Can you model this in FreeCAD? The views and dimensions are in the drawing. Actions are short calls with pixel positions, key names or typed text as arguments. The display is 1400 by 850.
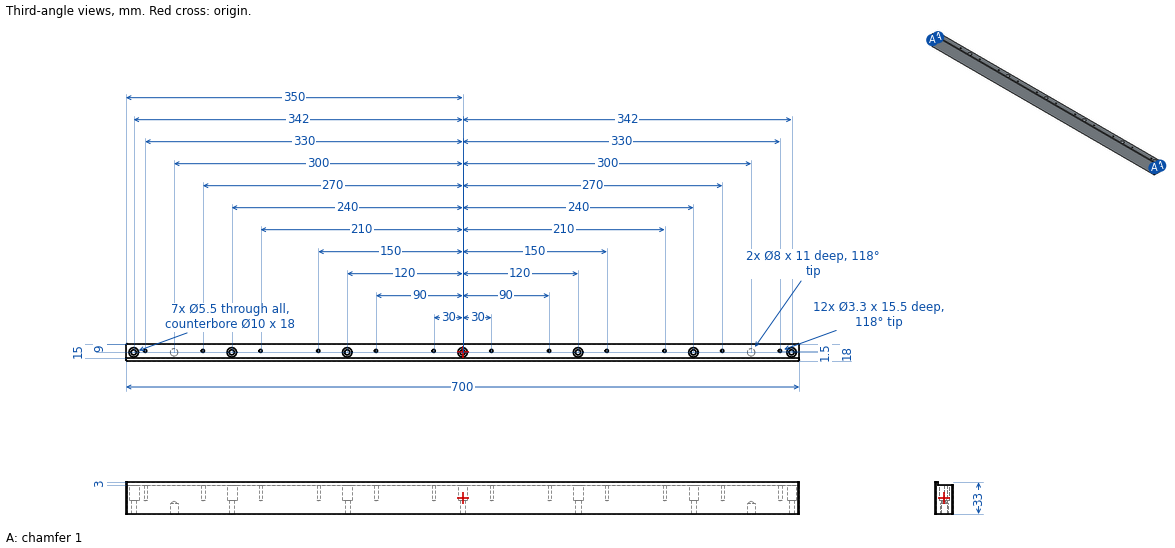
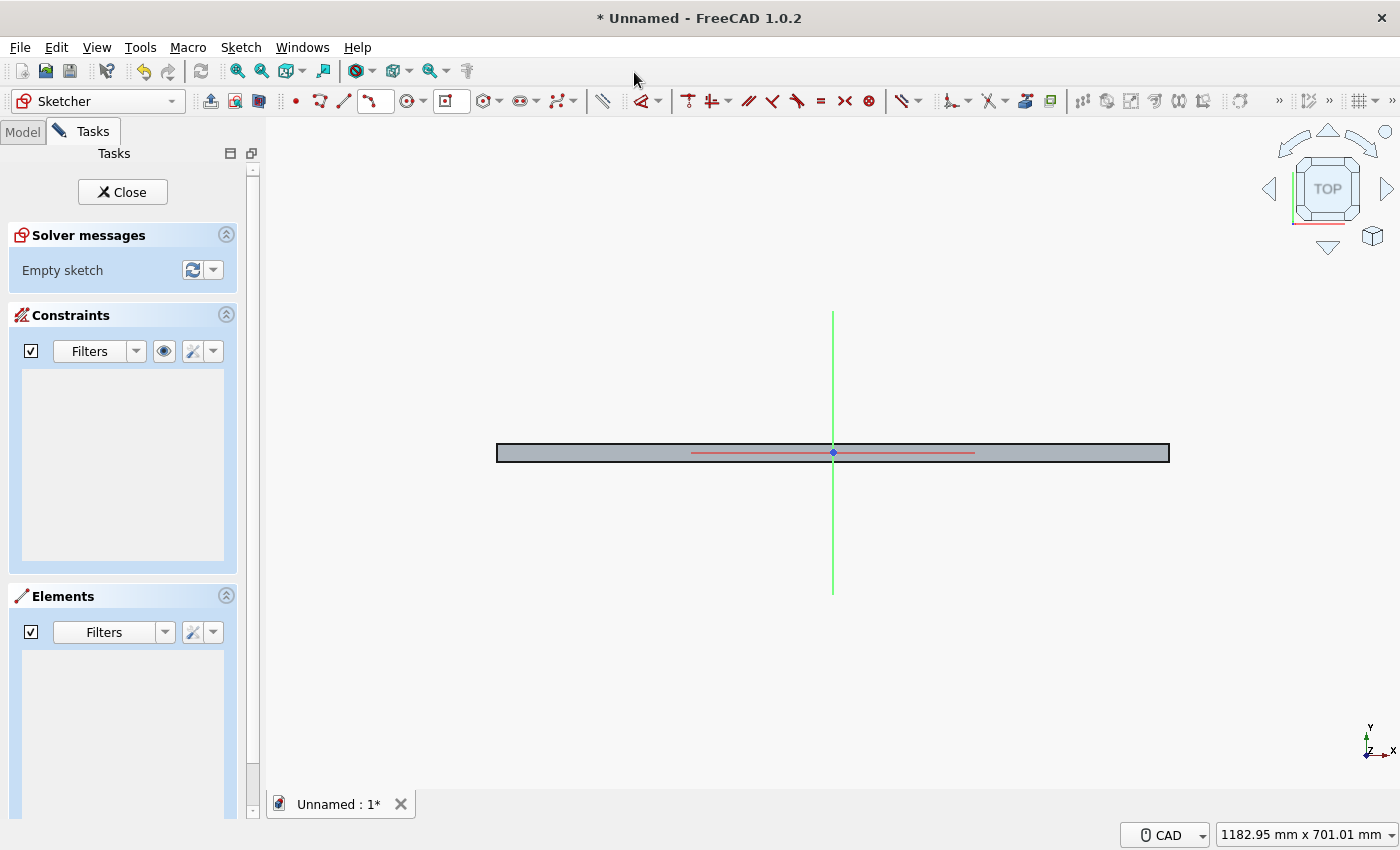
key(g)
key(r)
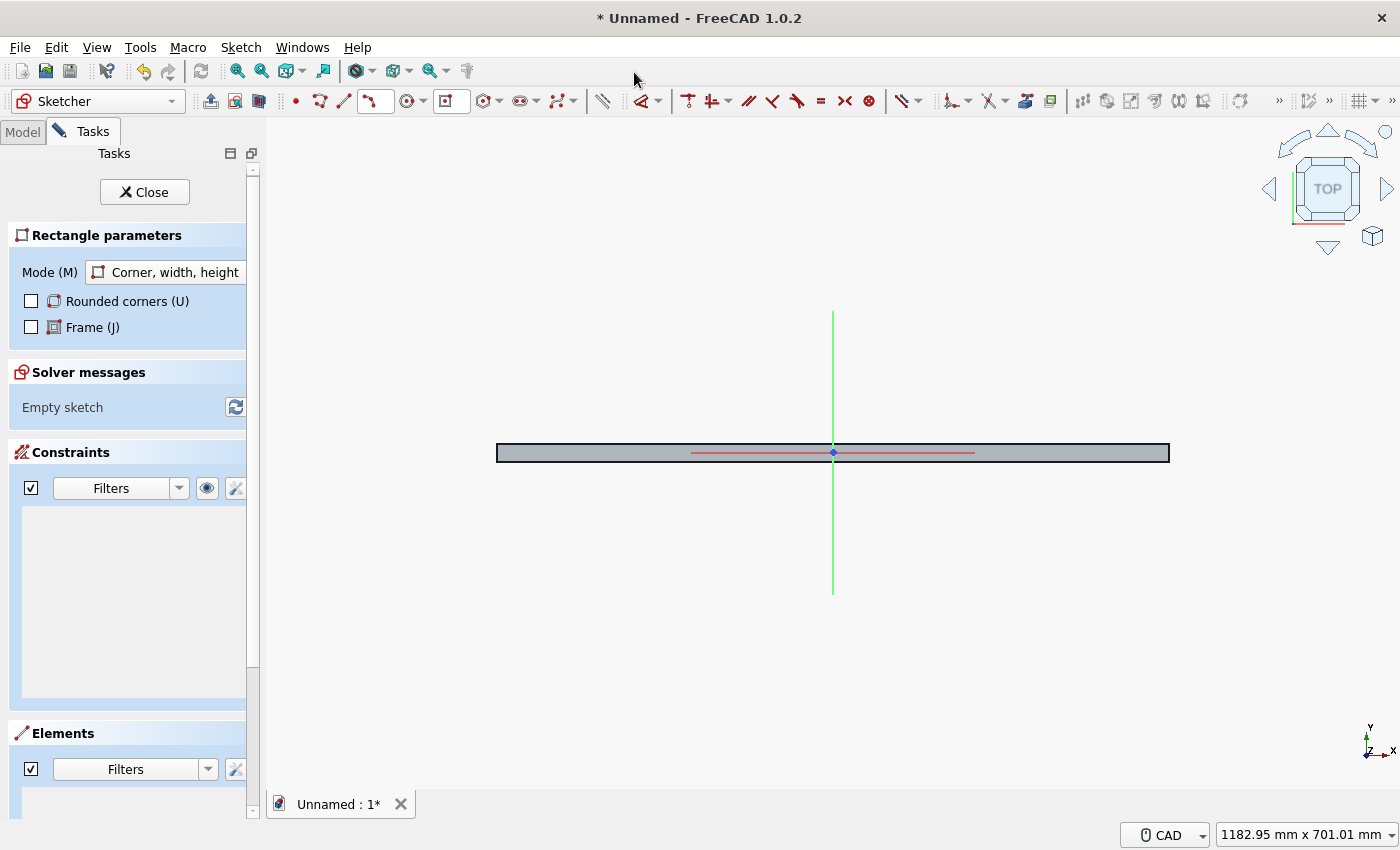
scroll(497, 444, up, 4)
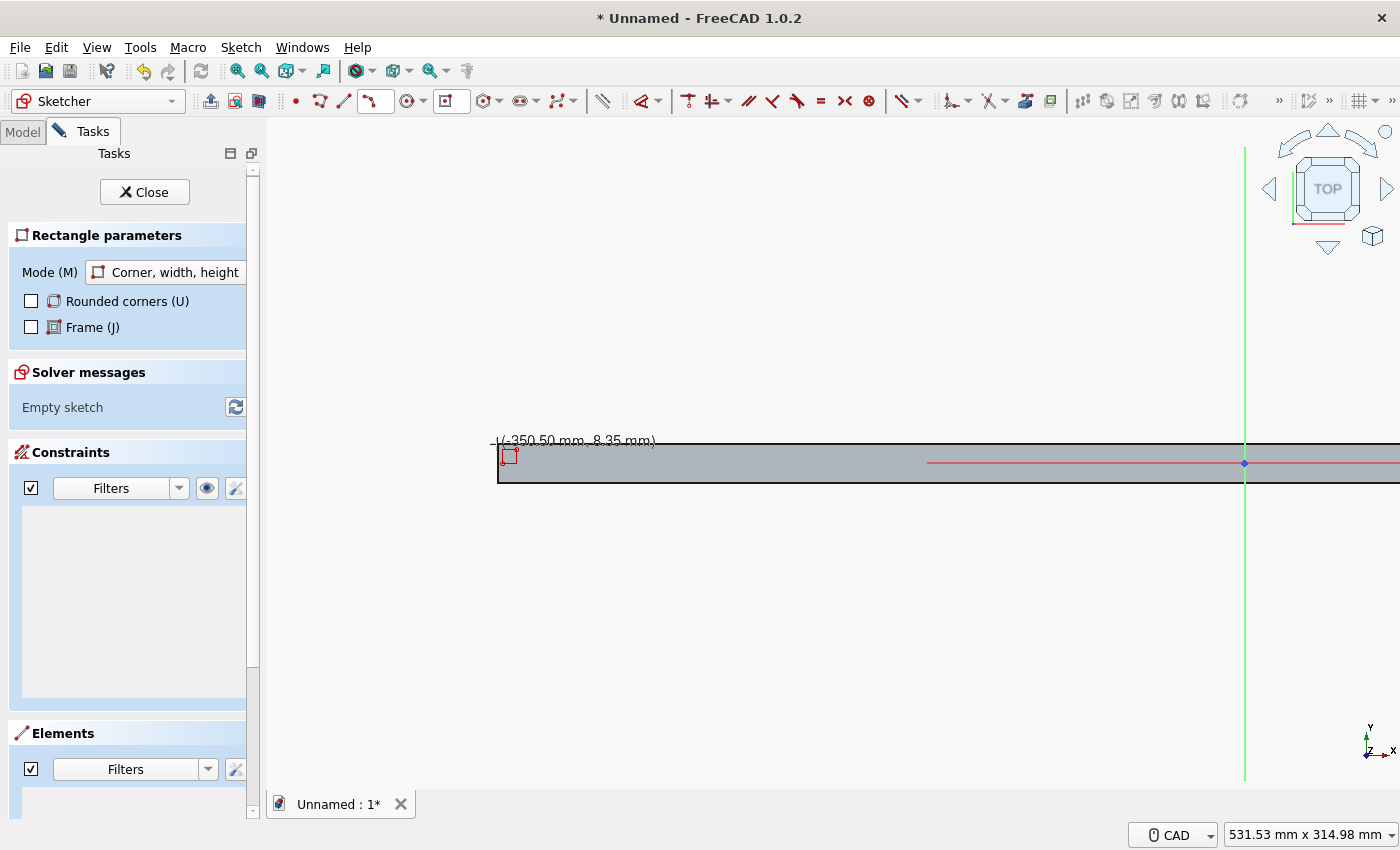
click(498, 444)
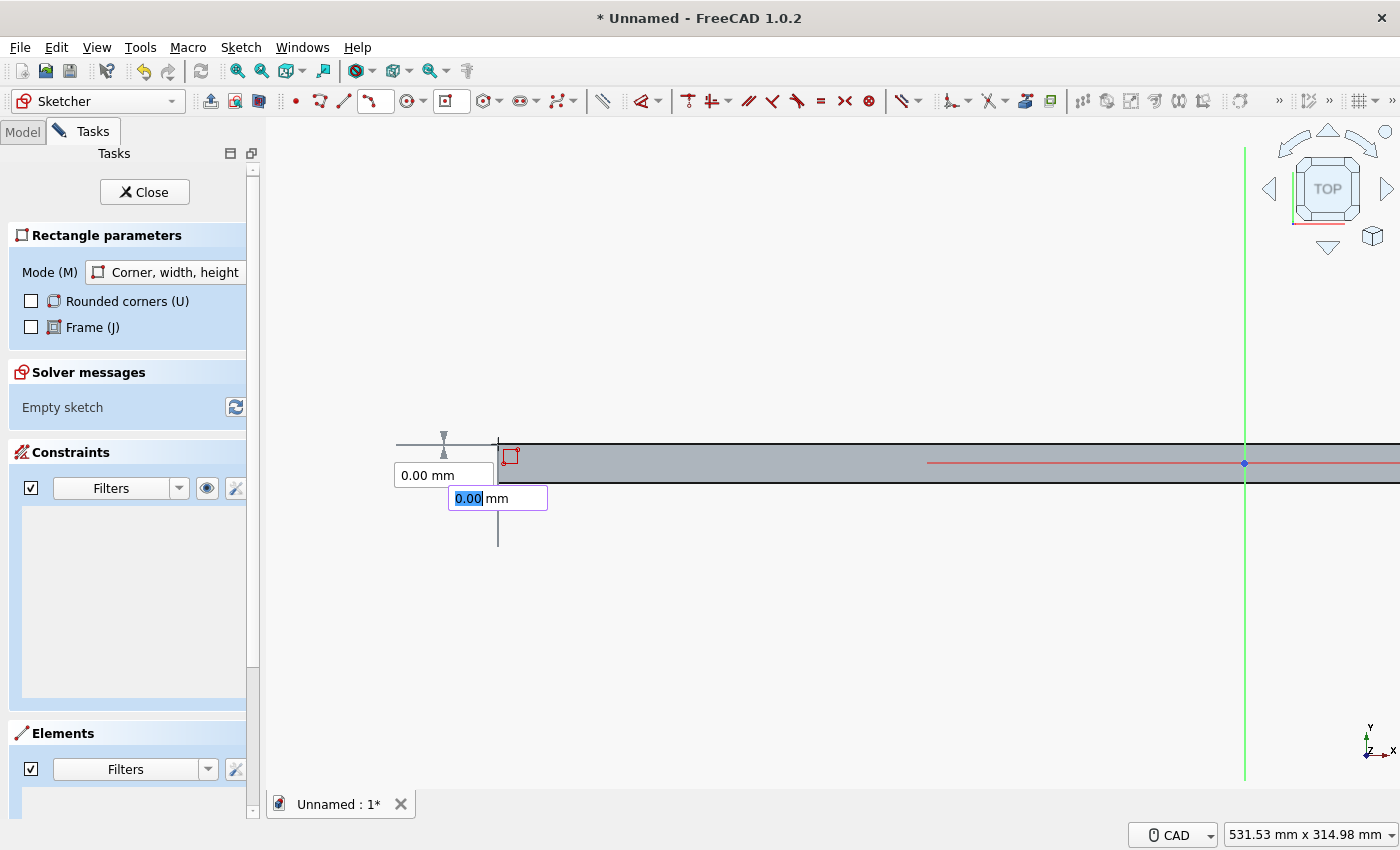
scroll(373, 447, down, 4)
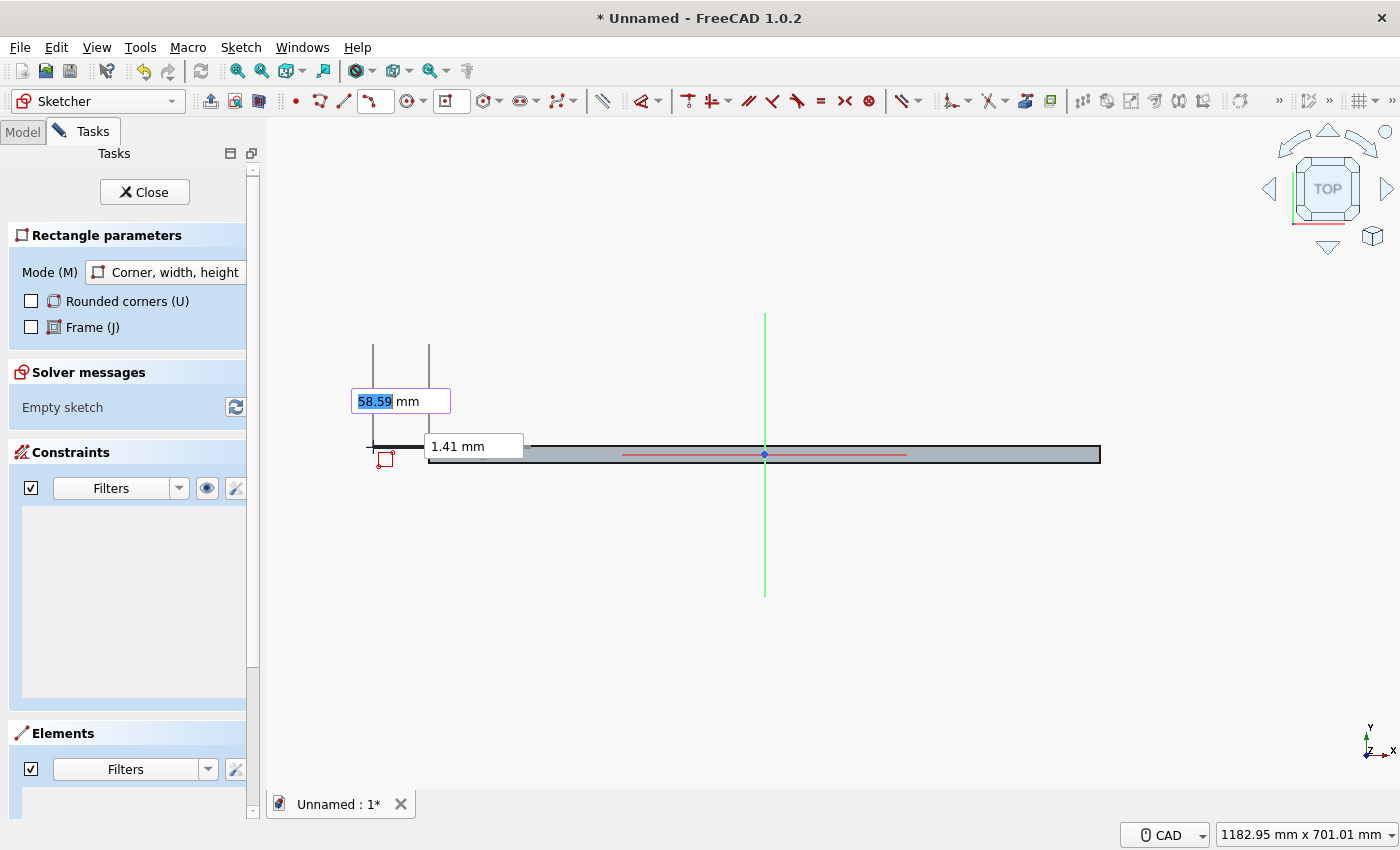
scroll(1100, 460, up, 6)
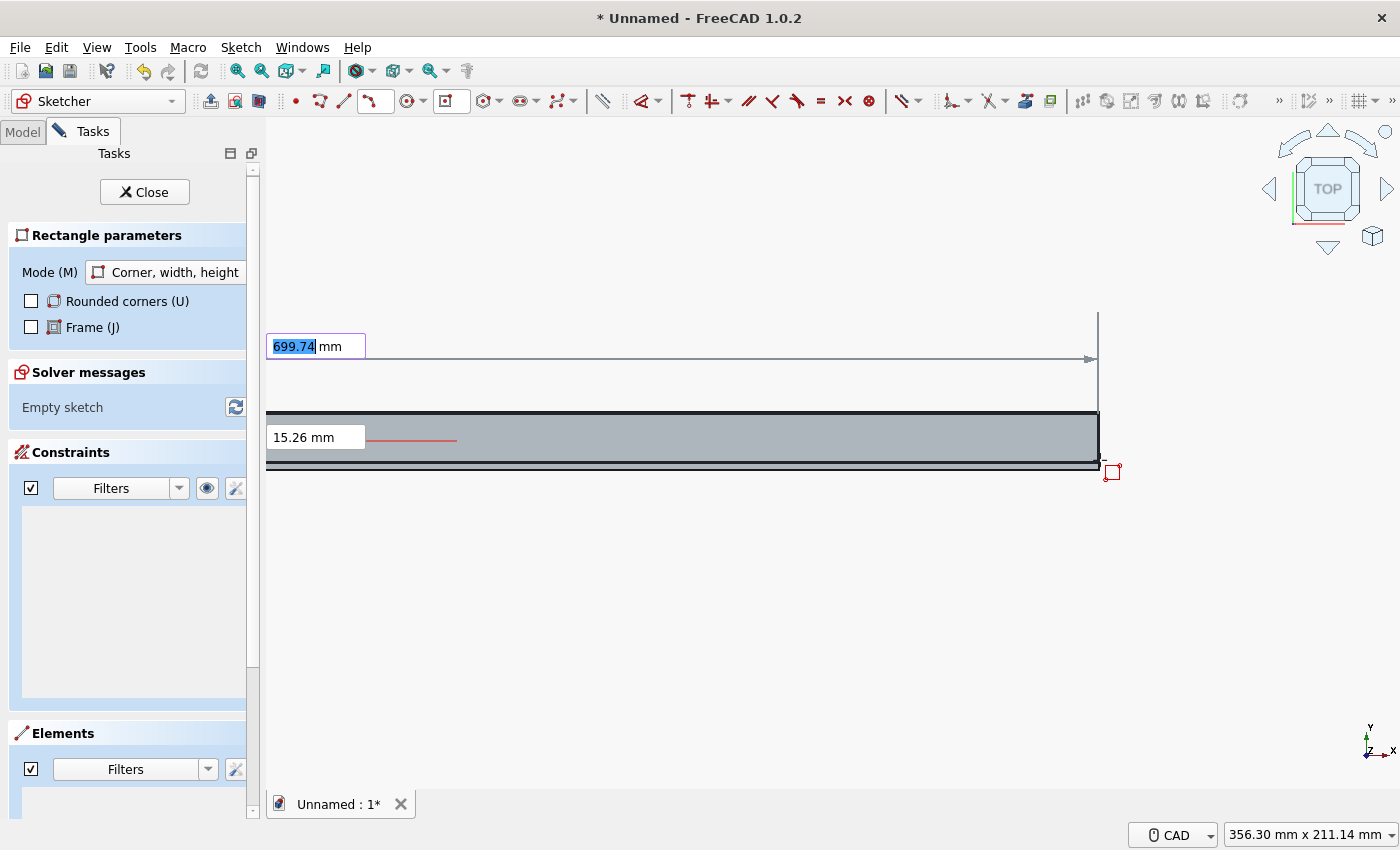
click(1099, 460)
key(Escape)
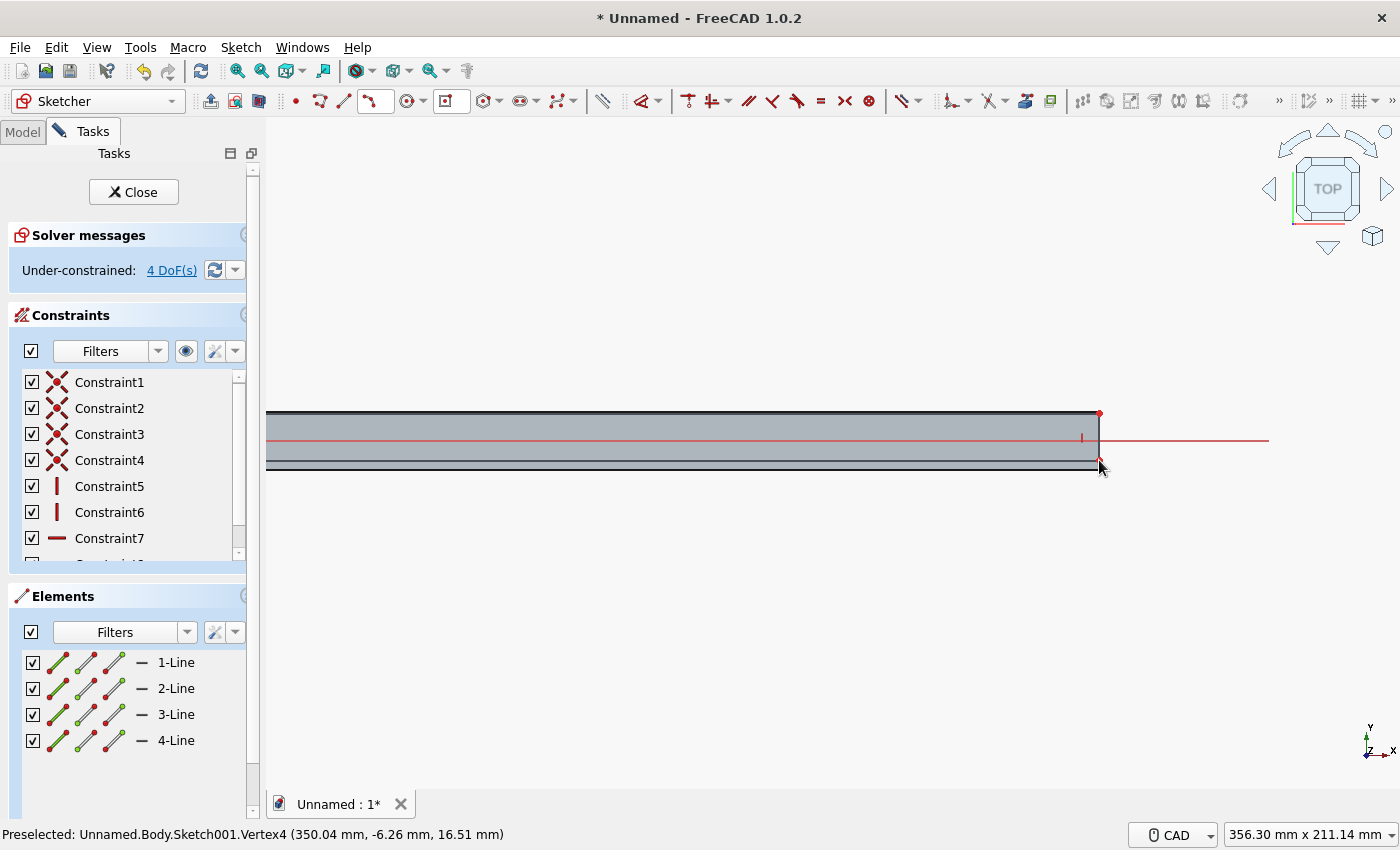
key(d)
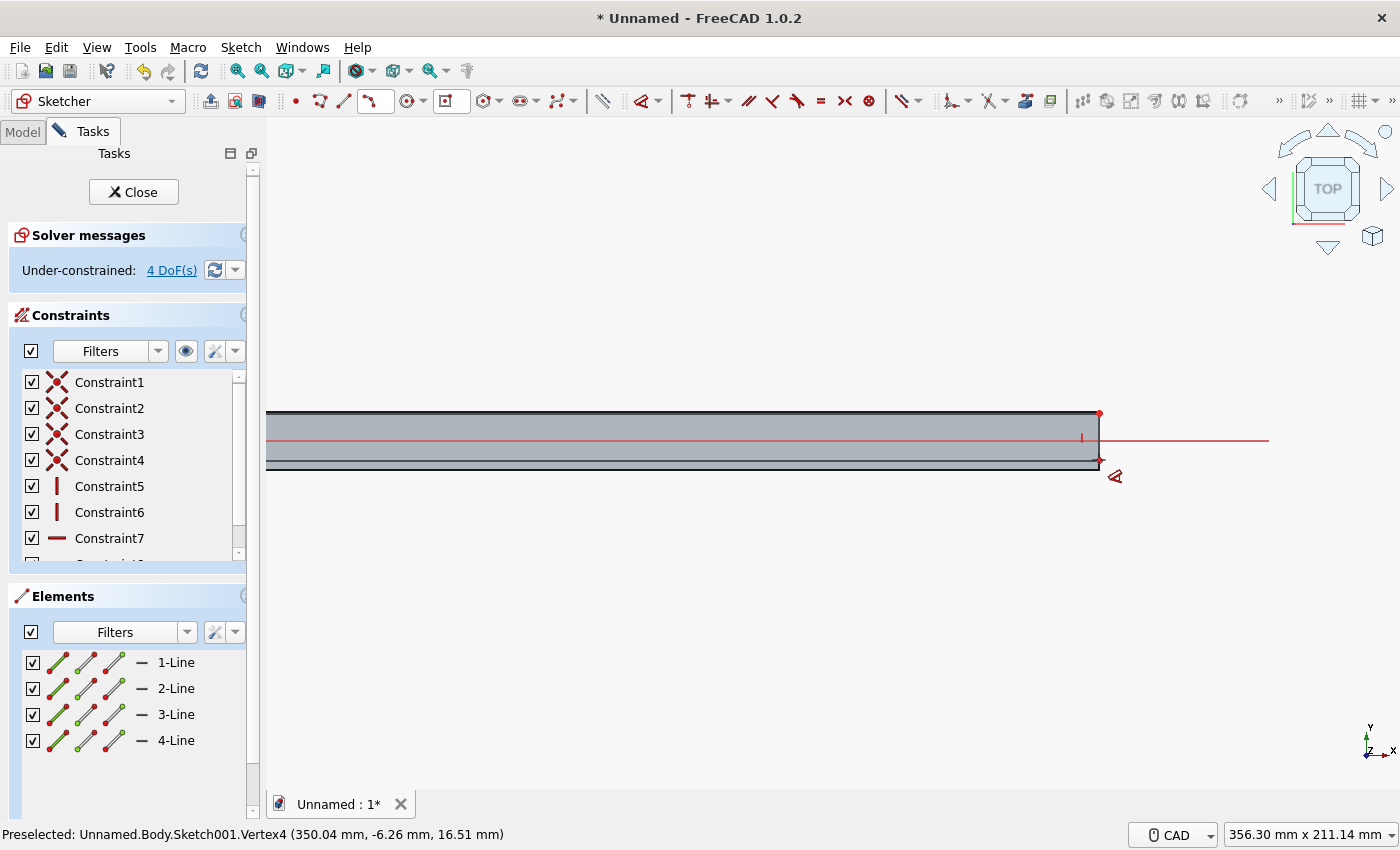
scroll(1101, 460, down, 6)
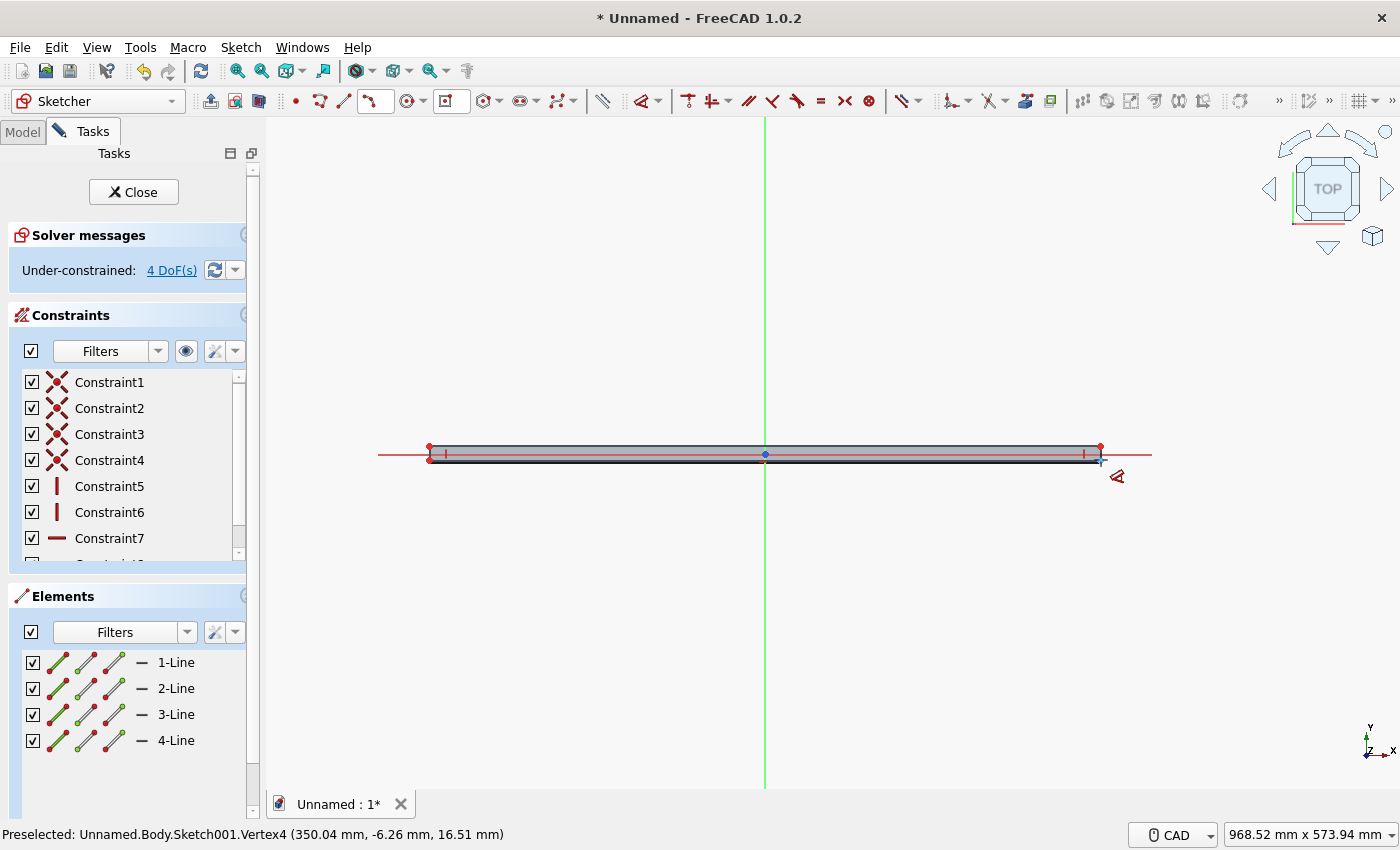
scroll(430, 451, up, 7)